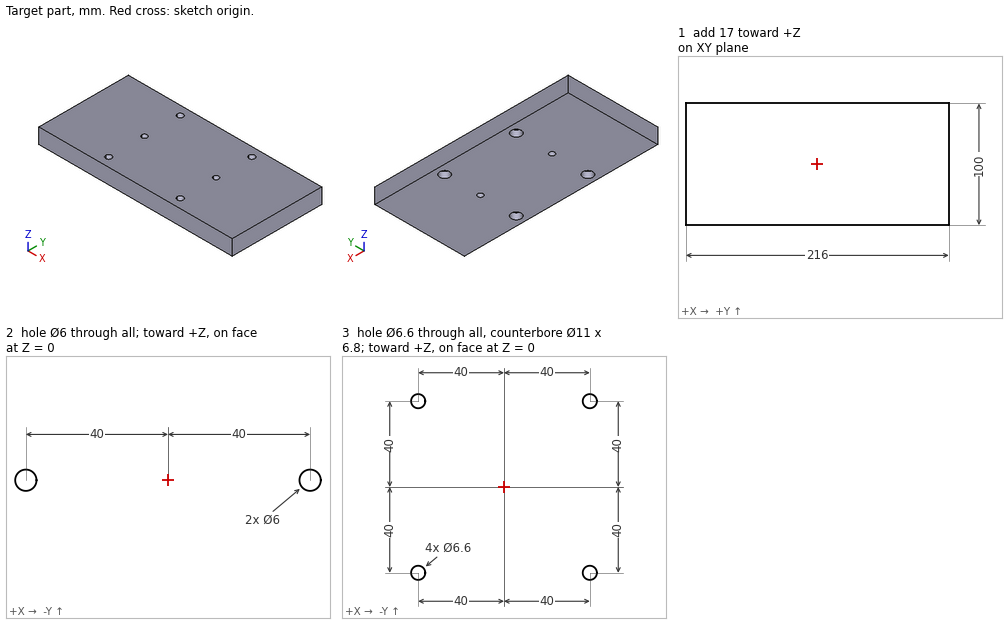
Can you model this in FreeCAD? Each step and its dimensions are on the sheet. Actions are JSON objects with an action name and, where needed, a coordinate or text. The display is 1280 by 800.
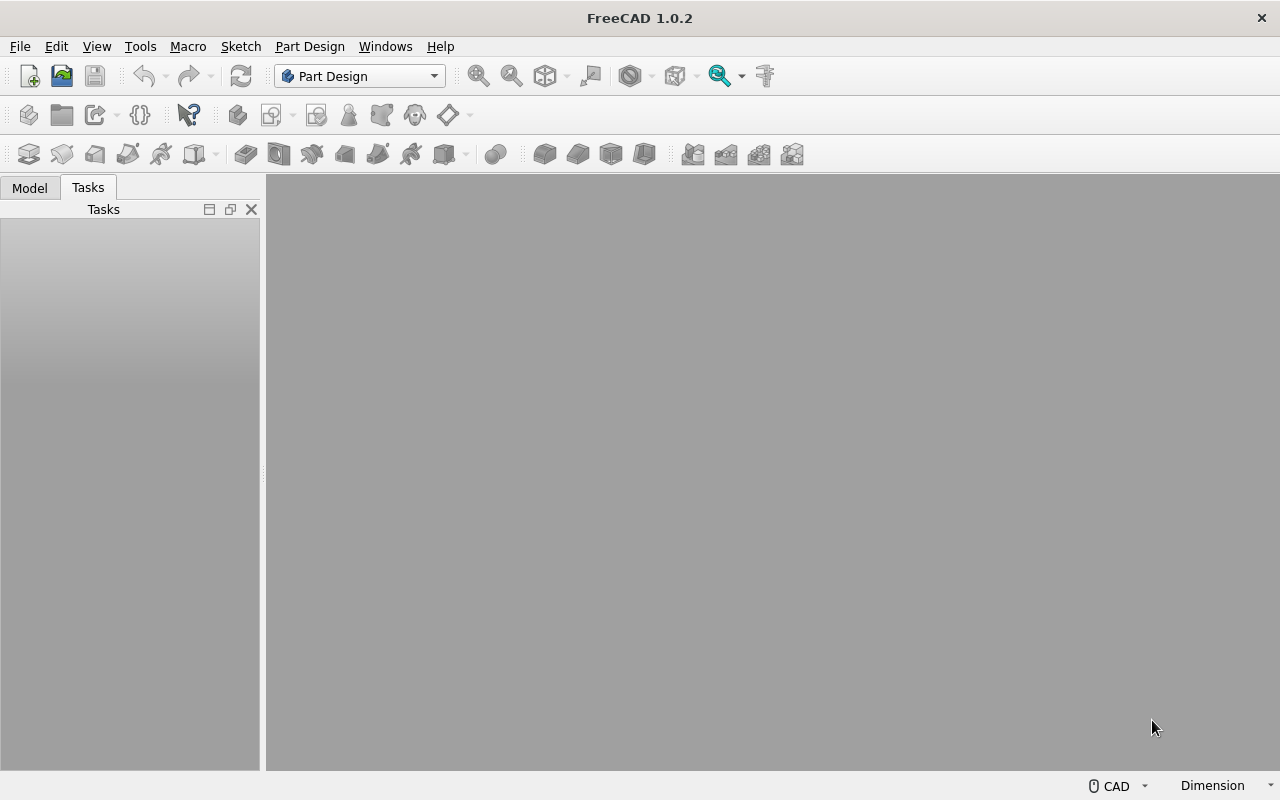
{"action": "left_click", "coordinate": [29, 76]}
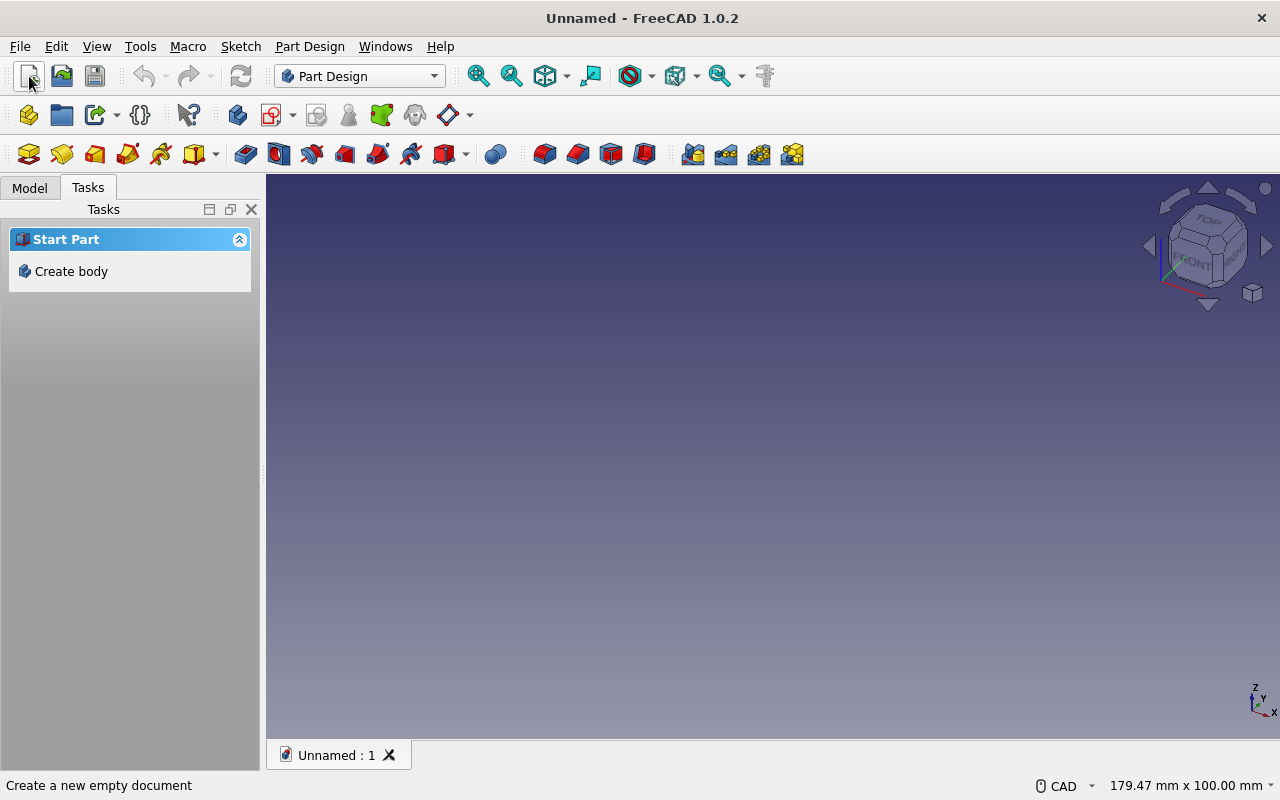
{"action": "left_click", "coordinate": [270, 116]}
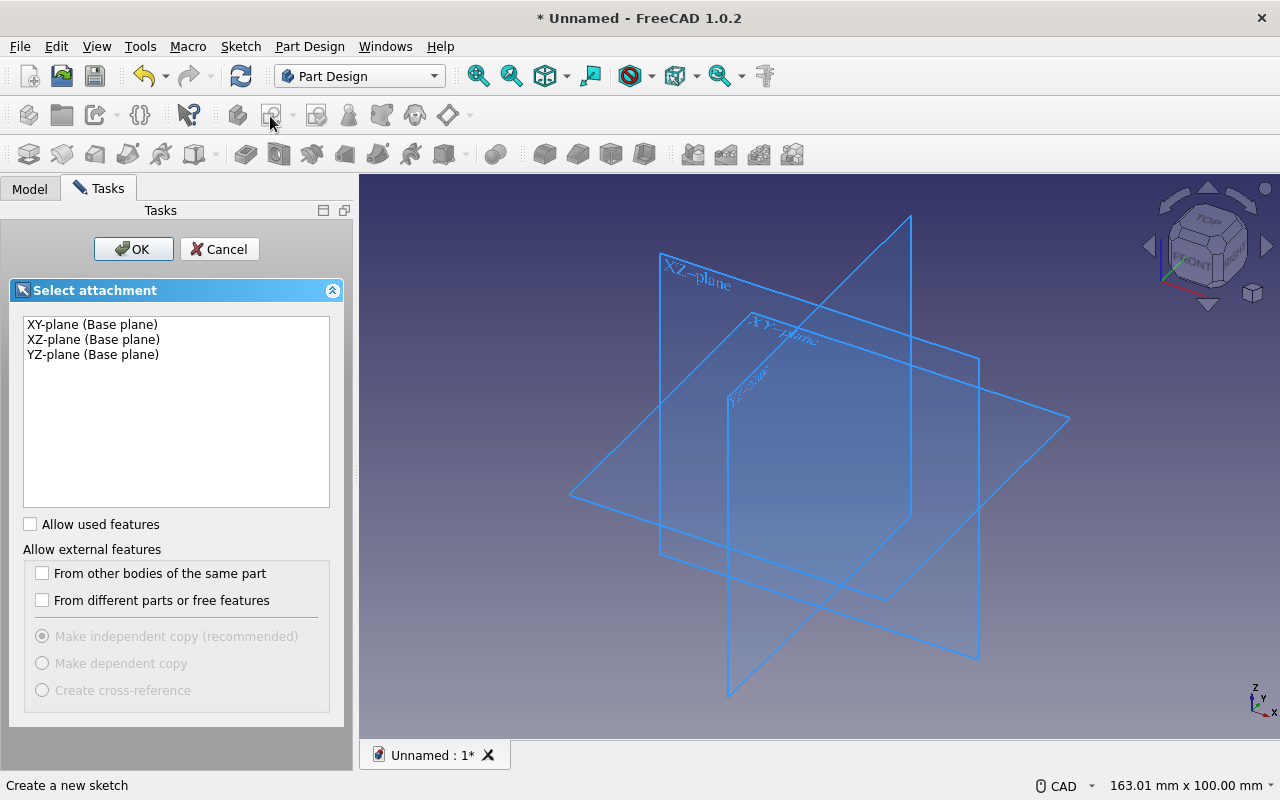
{"action": "left_click", "coordinate": [84, 324]}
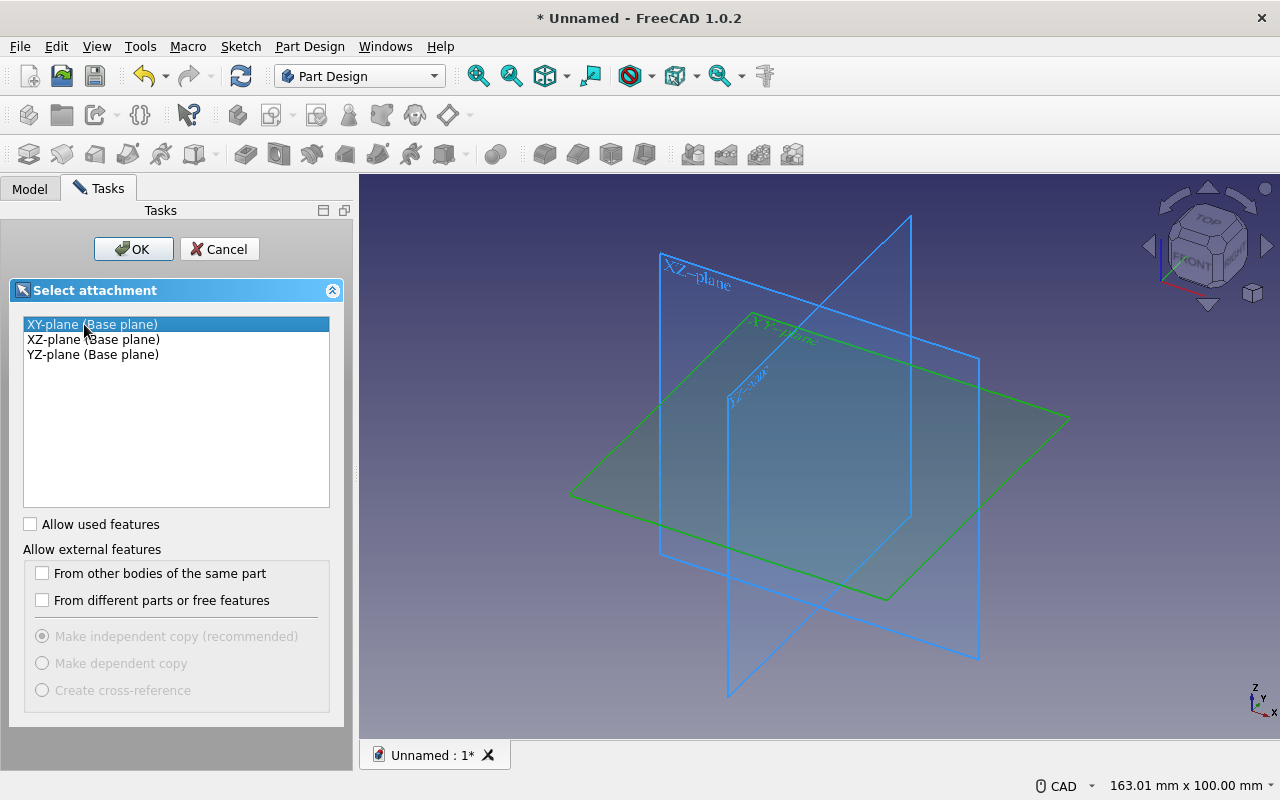
{"action": "left_click", "coordinate": [134, 249]}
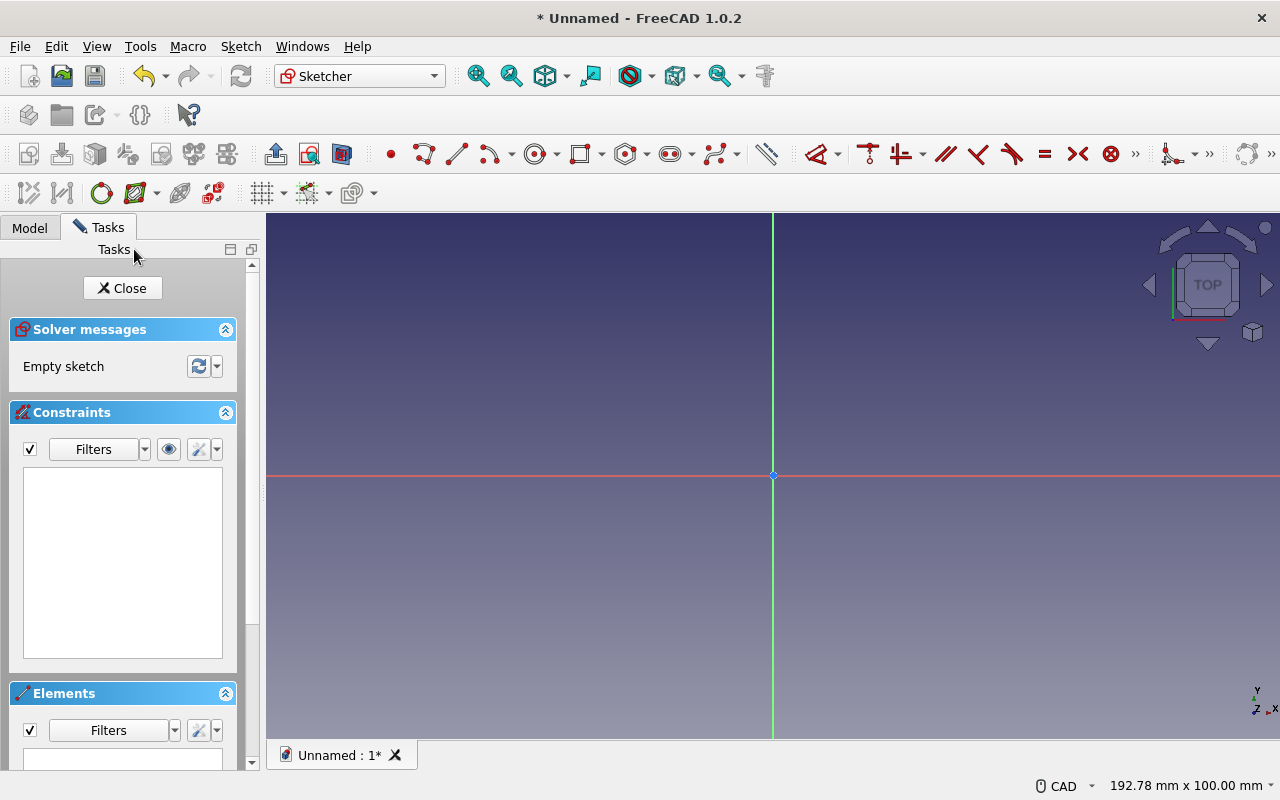
{"action": "scroll", "coordinate": [621, 476], "scroll_direction": "down", "scroll_amount": 3}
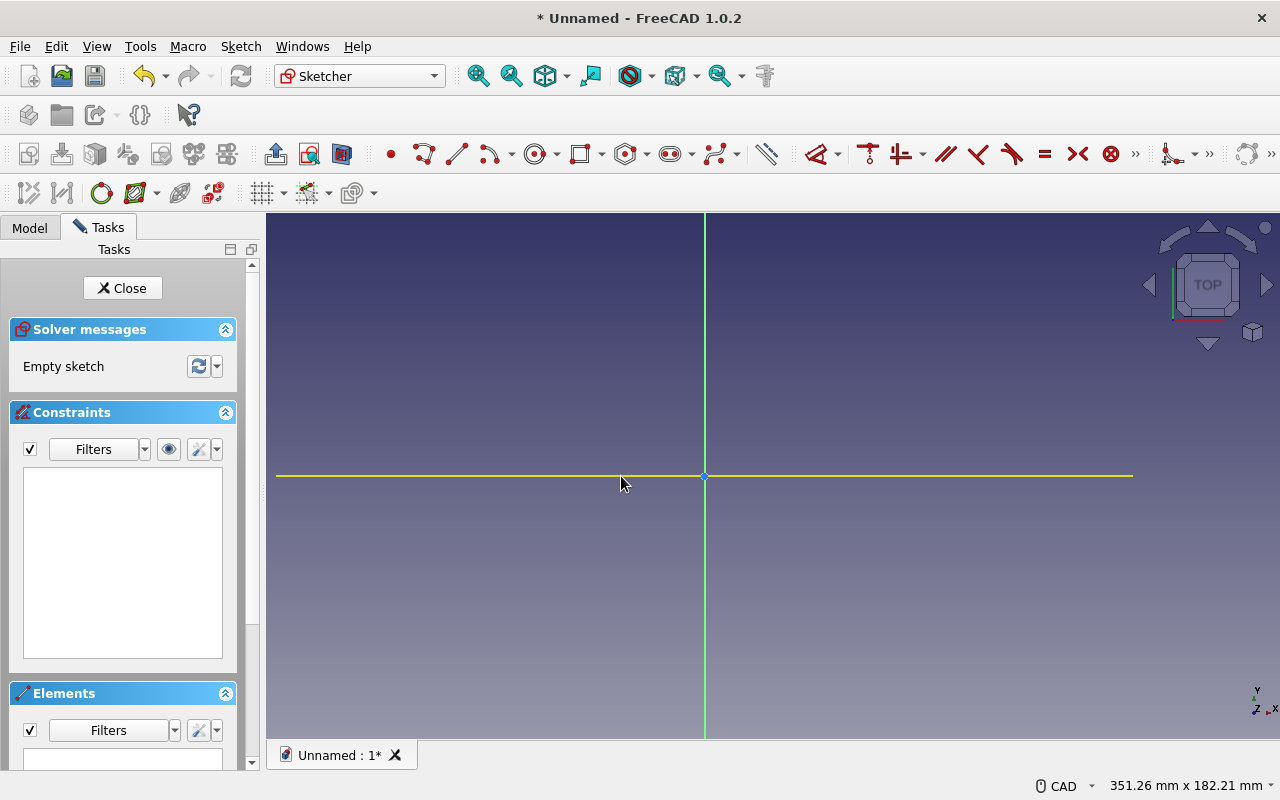
{"action": "left_click", "coordinate": [602, 154]}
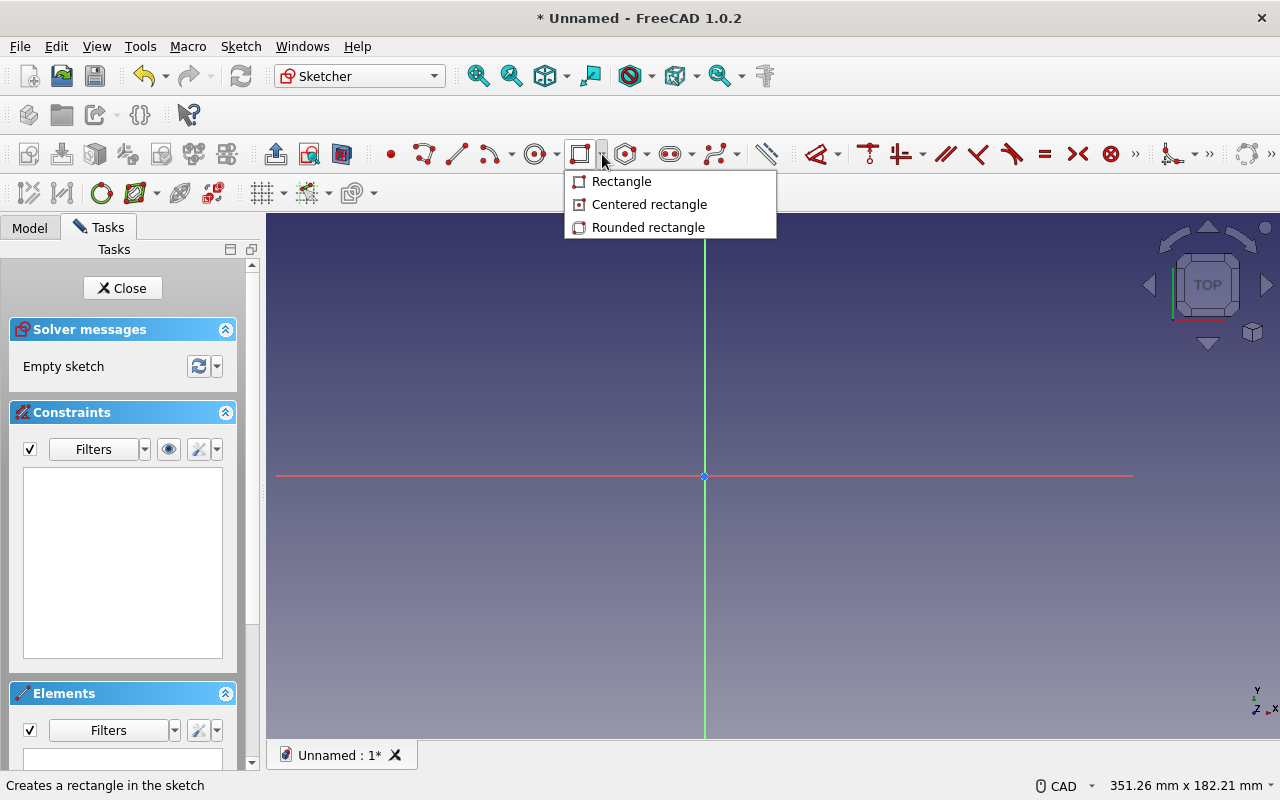
{"action": "left_click", "coordinate": [670, 204]}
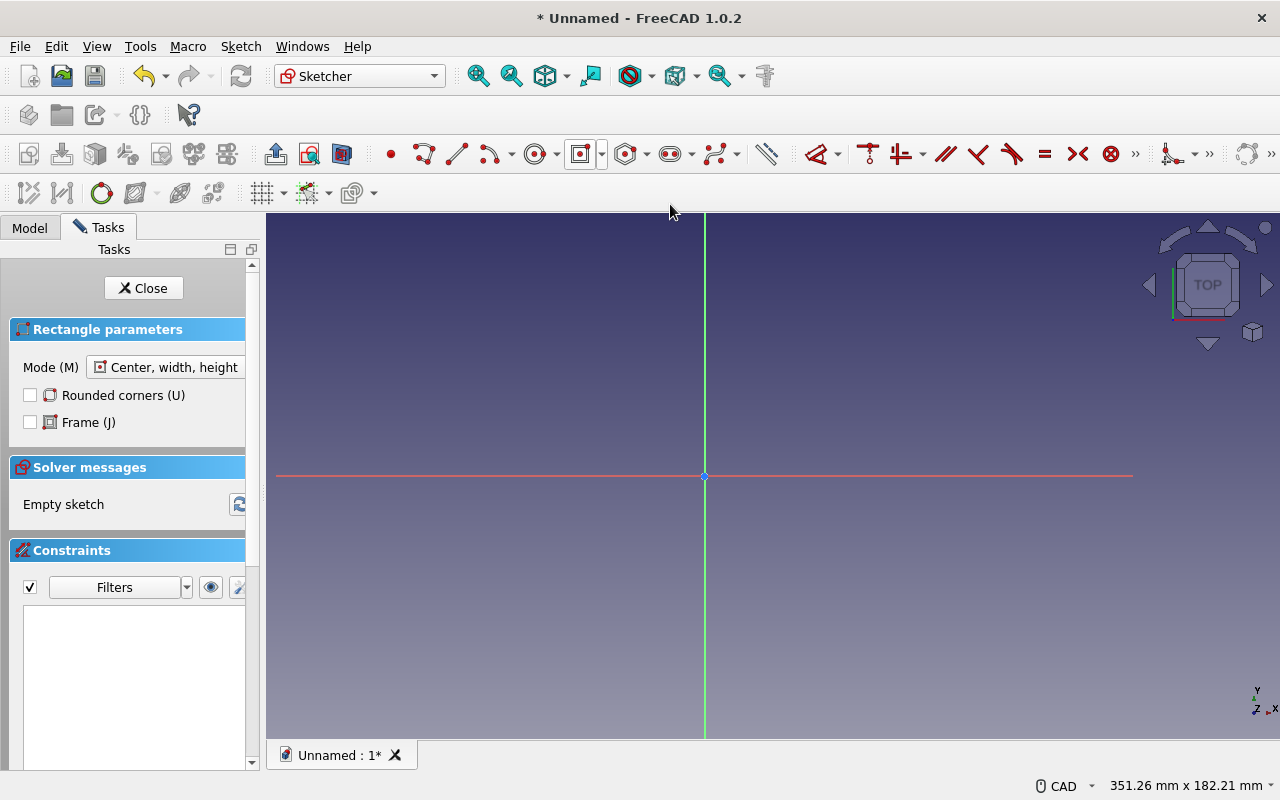
{"action": "left_click", "coordinate": [705, 476]}
{"action": "mouse_move", "coordinate": [1016, 332]}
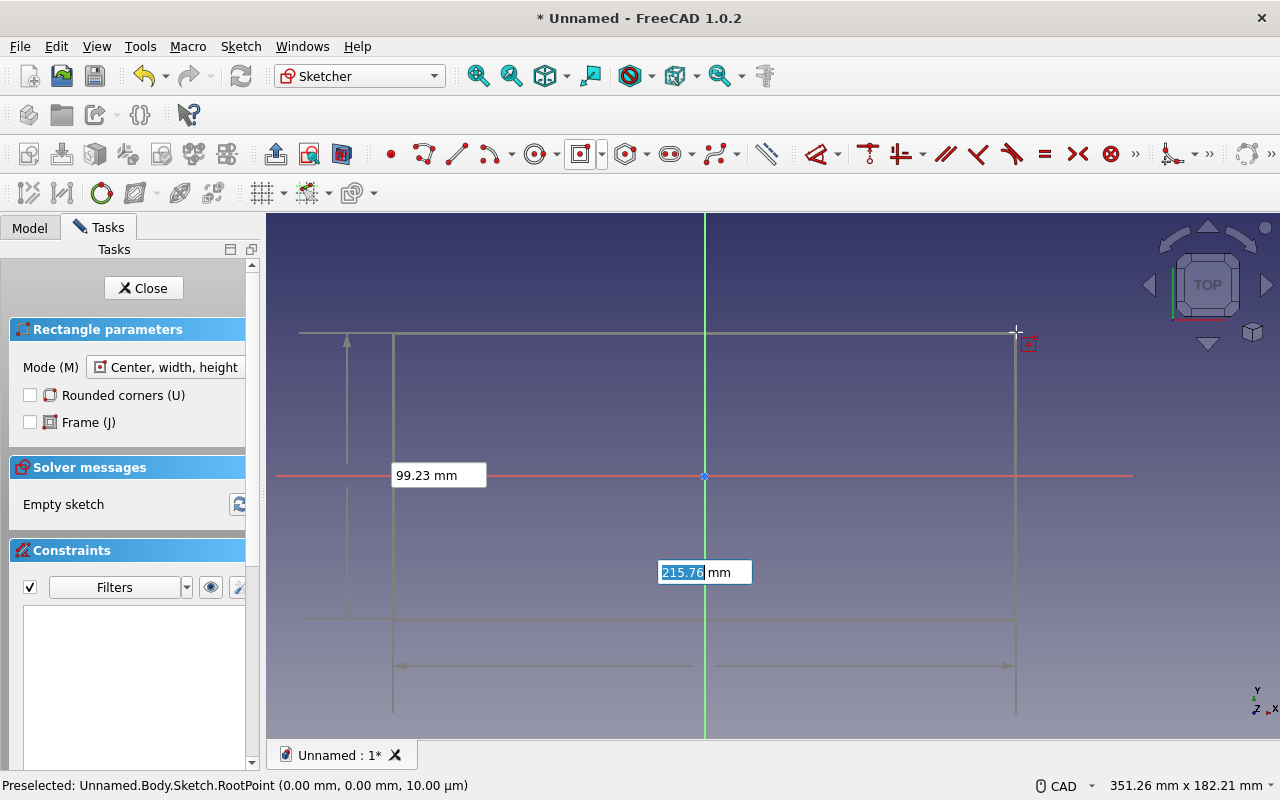
{"action": "type", "text": "216"}
{"action": "key", "text": "Tab"}
{"action": "type", "text": "100"}
{"action": "key", "text": "Return"}
{"action": "key", "text": "Escape"}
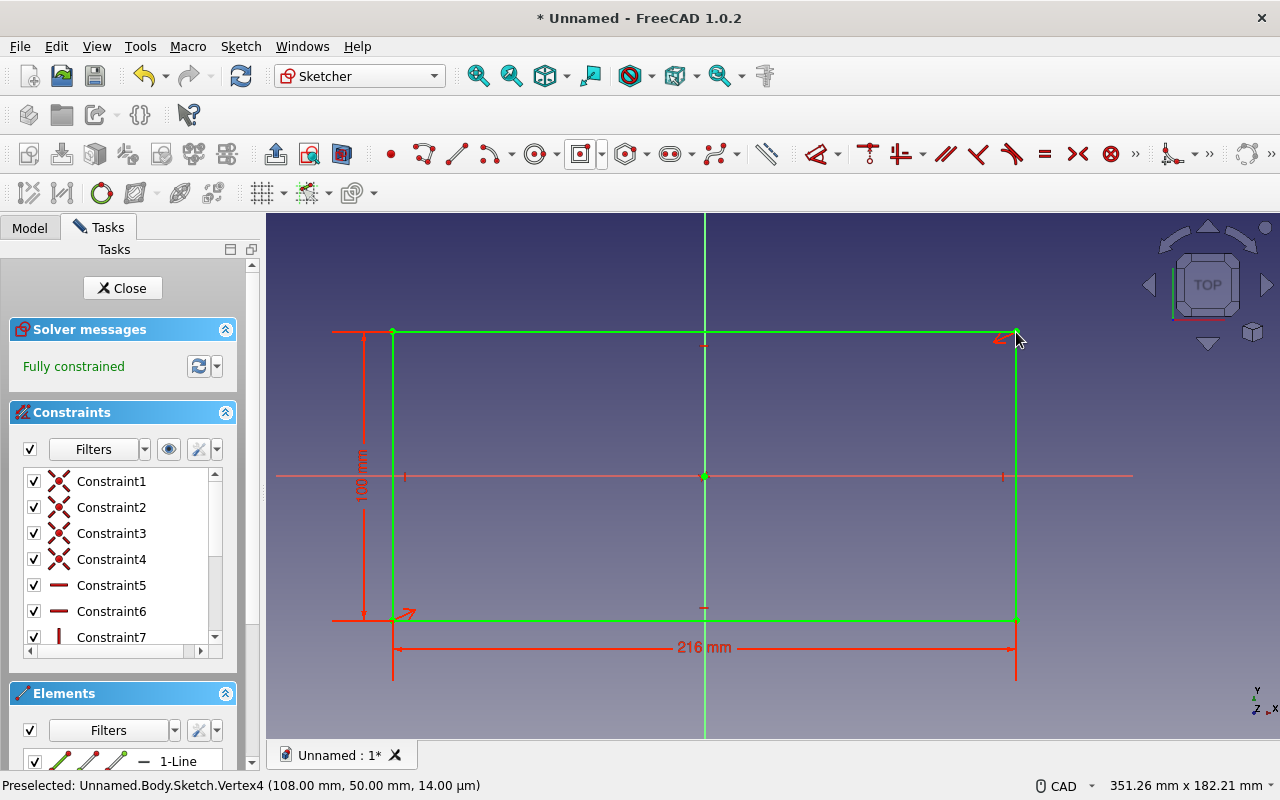
{"action": "left_click", "coordinate": [123, 288]}